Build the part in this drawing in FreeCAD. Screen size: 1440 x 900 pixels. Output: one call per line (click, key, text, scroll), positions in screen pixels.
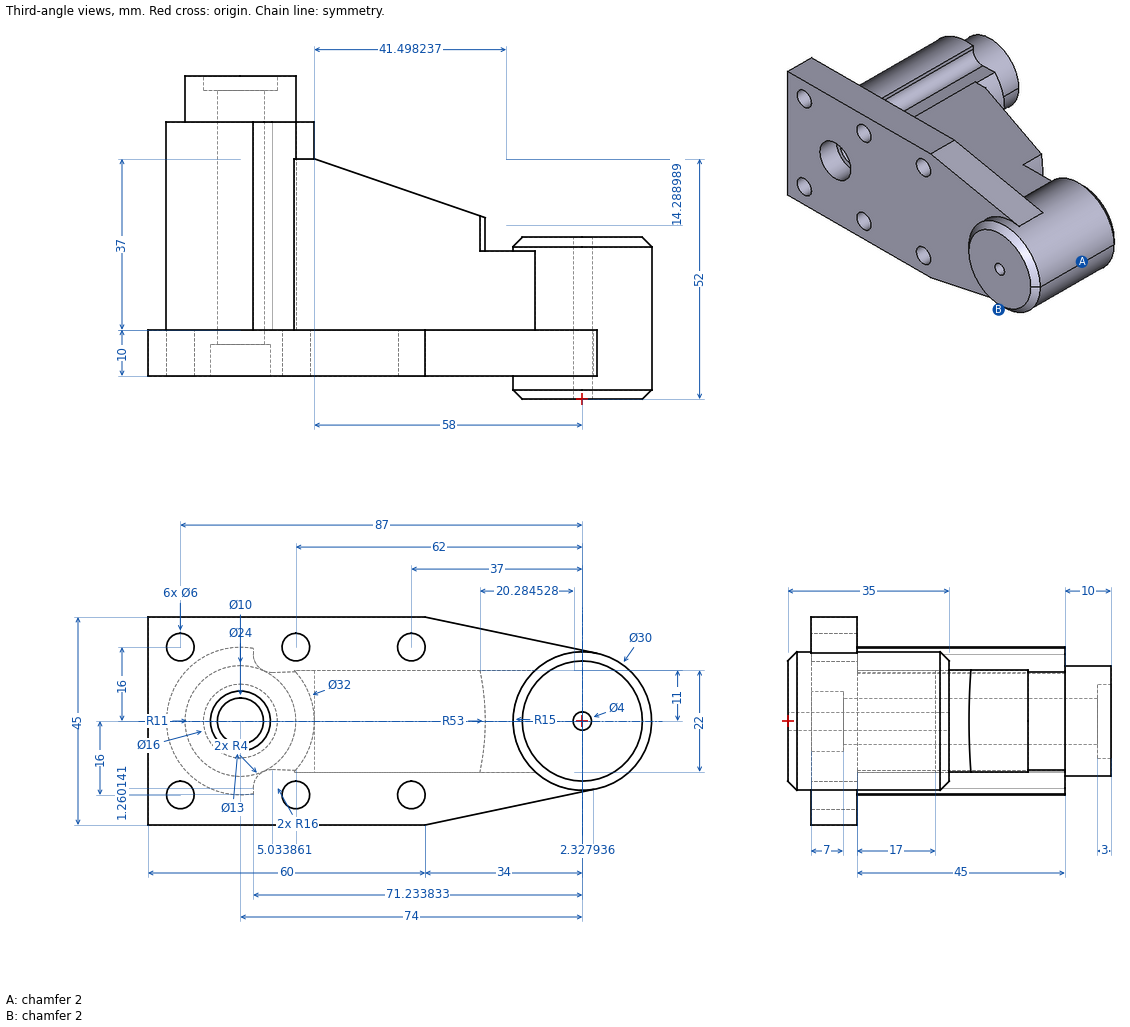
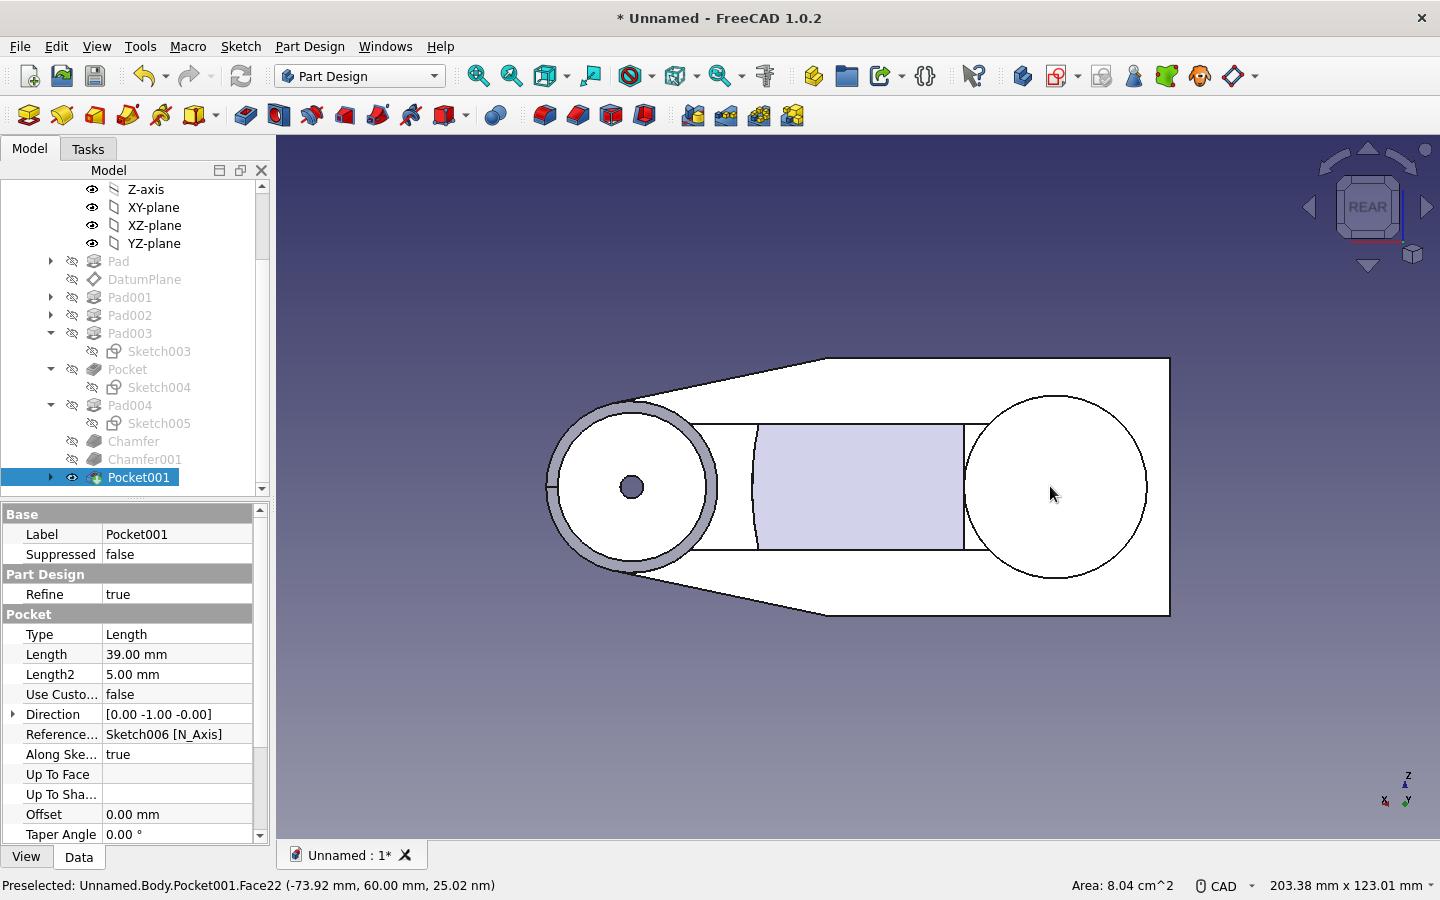
click(1056, 76)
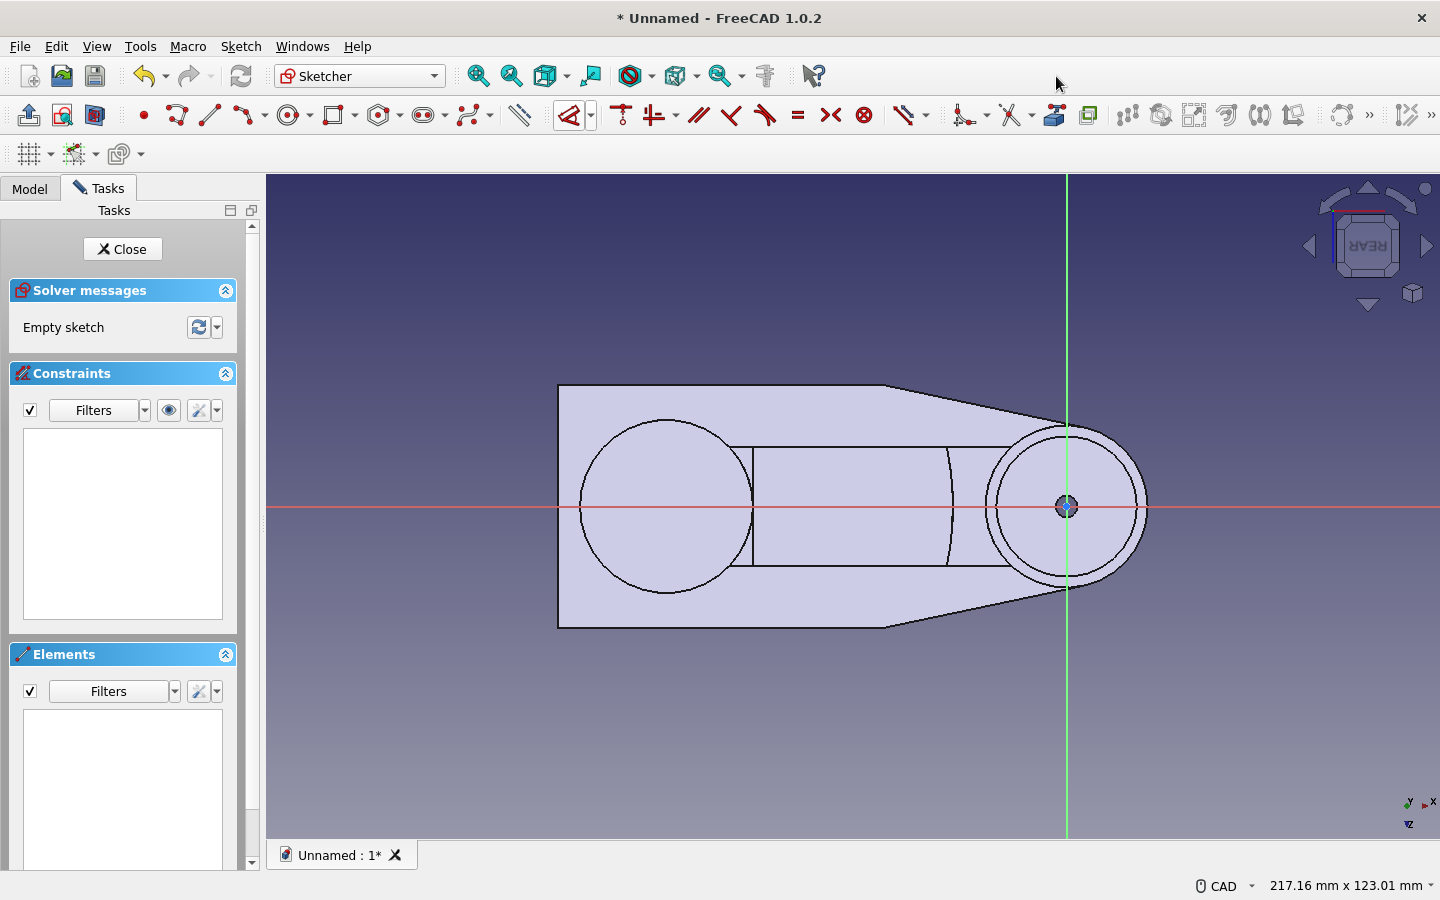
scroll(616, 506, up, 6)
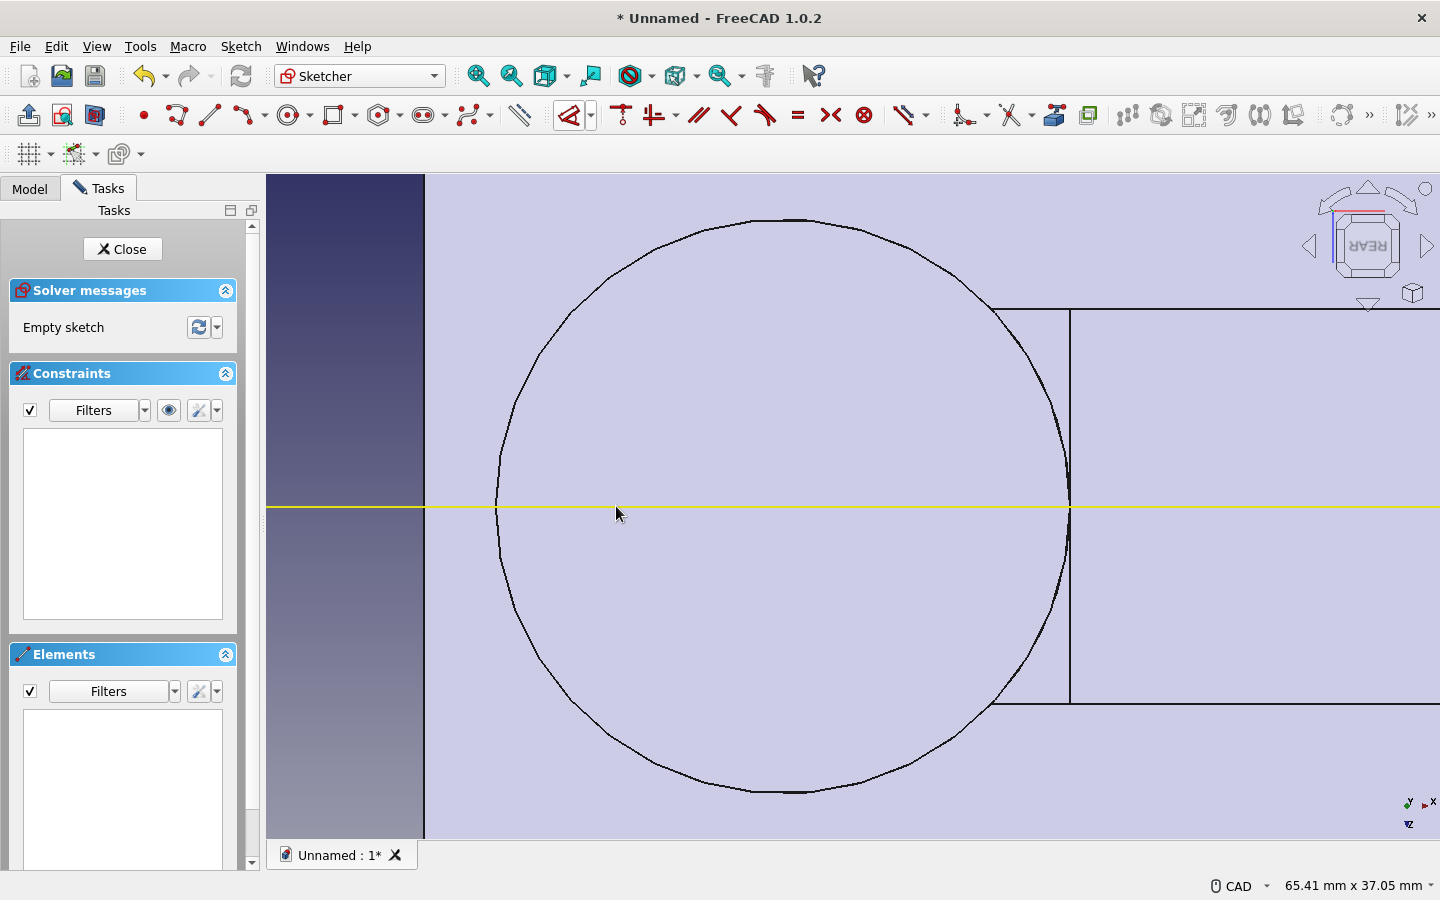
click(288, 116)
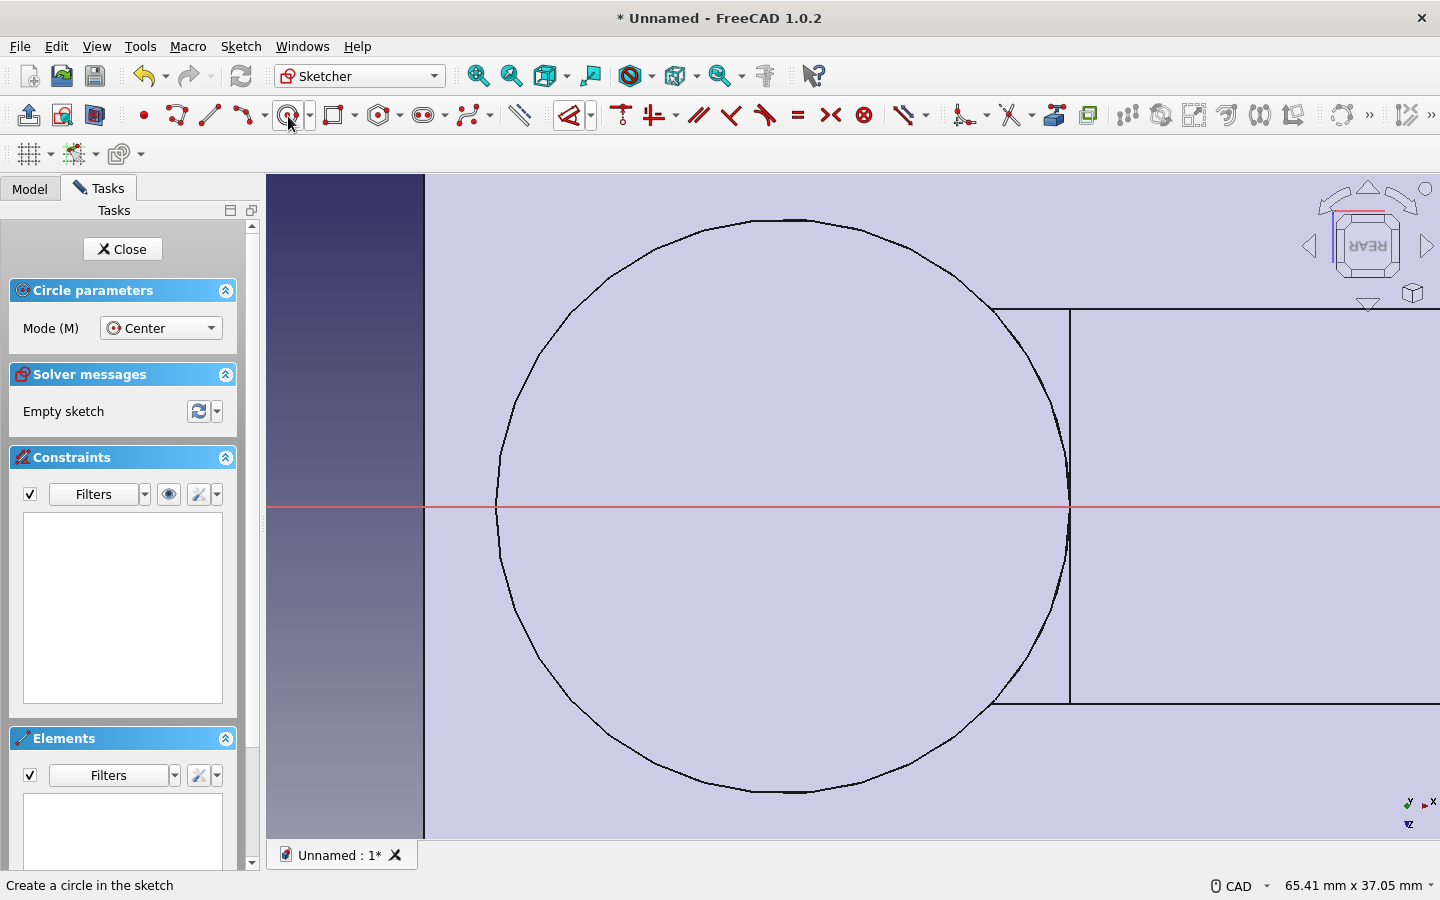
click(783, 506)
click(935, 354)
key(Escape)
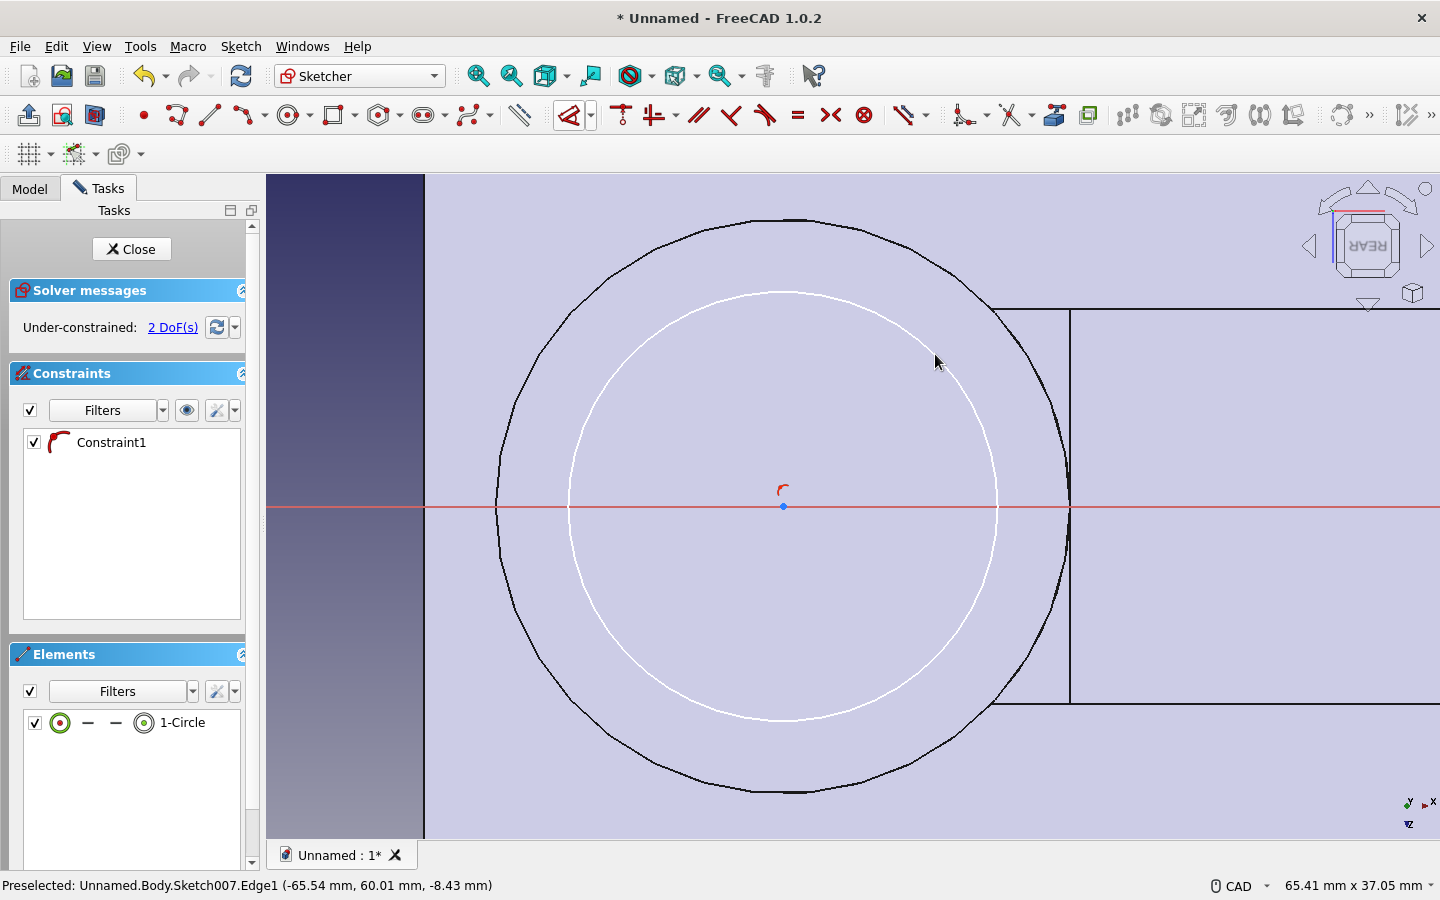
click(934, 354)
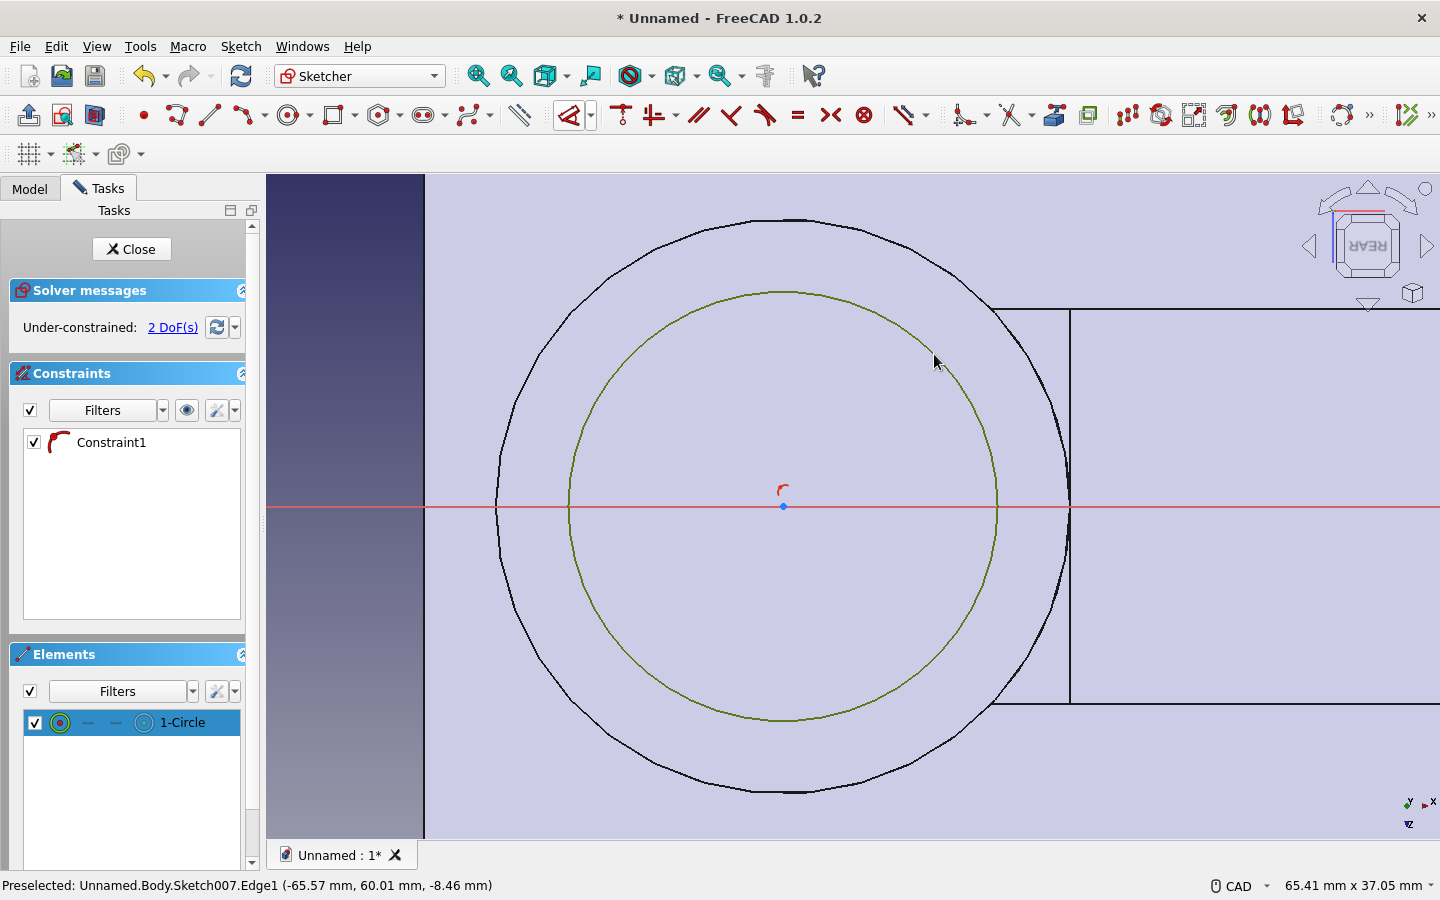
key(k)
key(o)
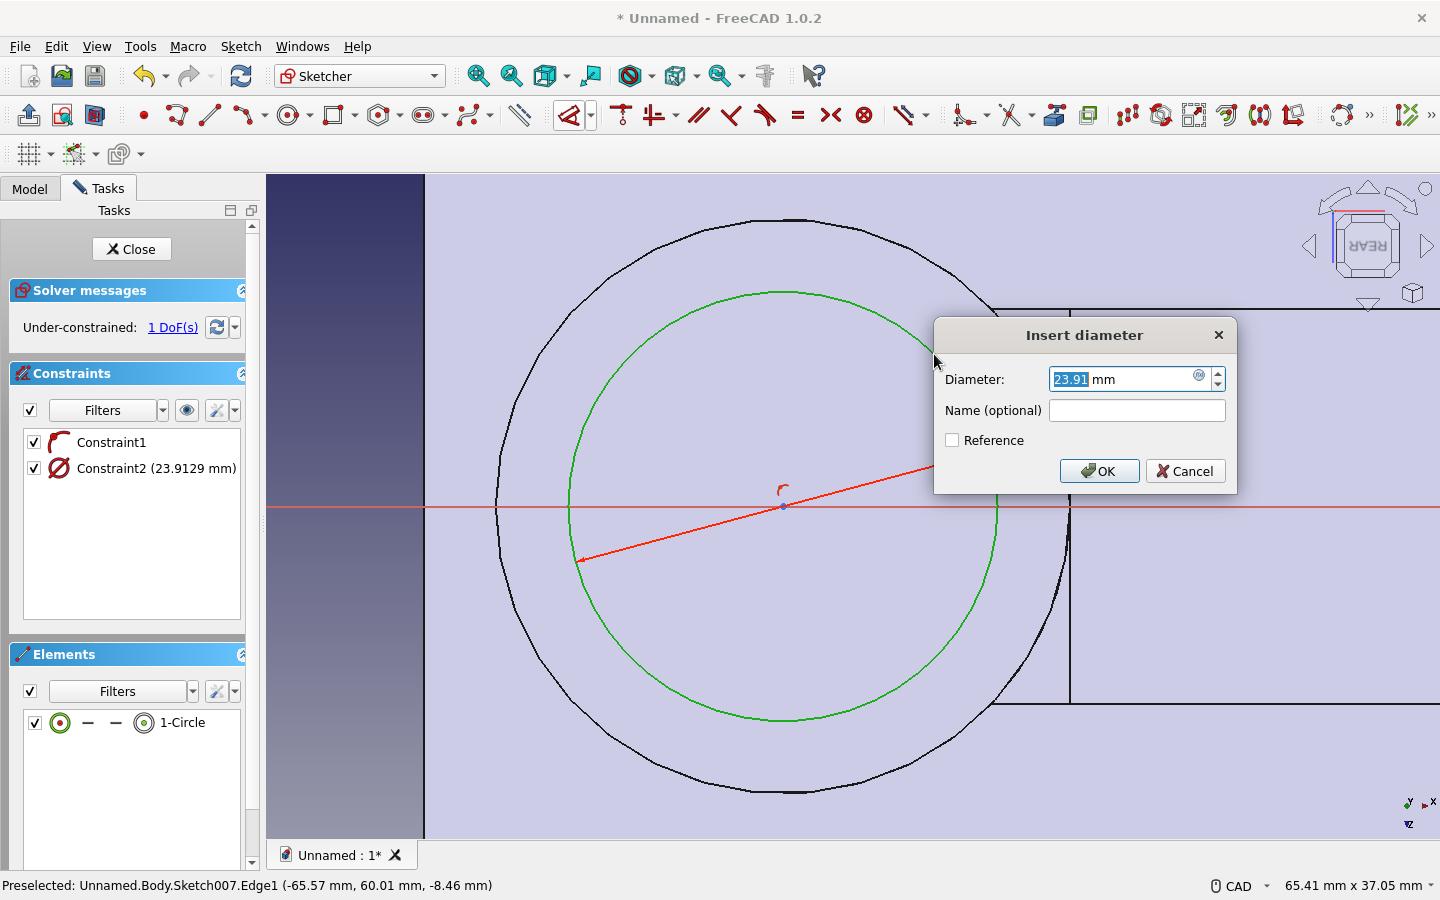
text(24)
key(Return)